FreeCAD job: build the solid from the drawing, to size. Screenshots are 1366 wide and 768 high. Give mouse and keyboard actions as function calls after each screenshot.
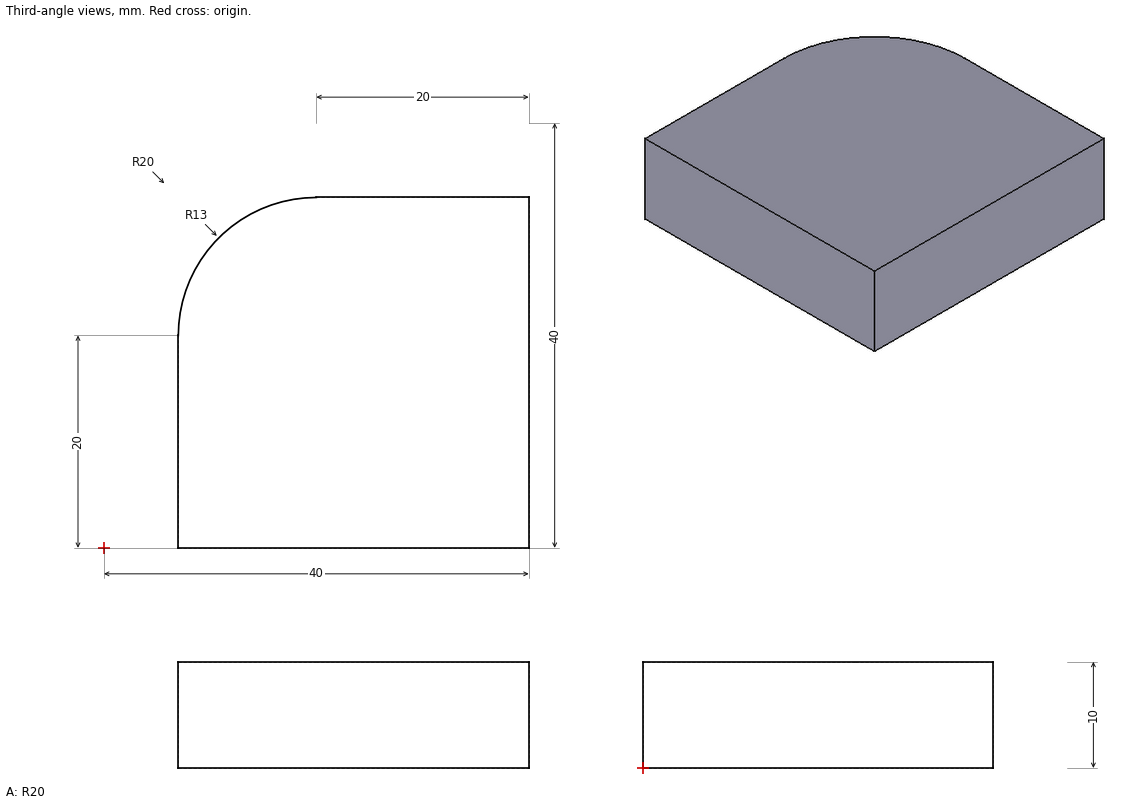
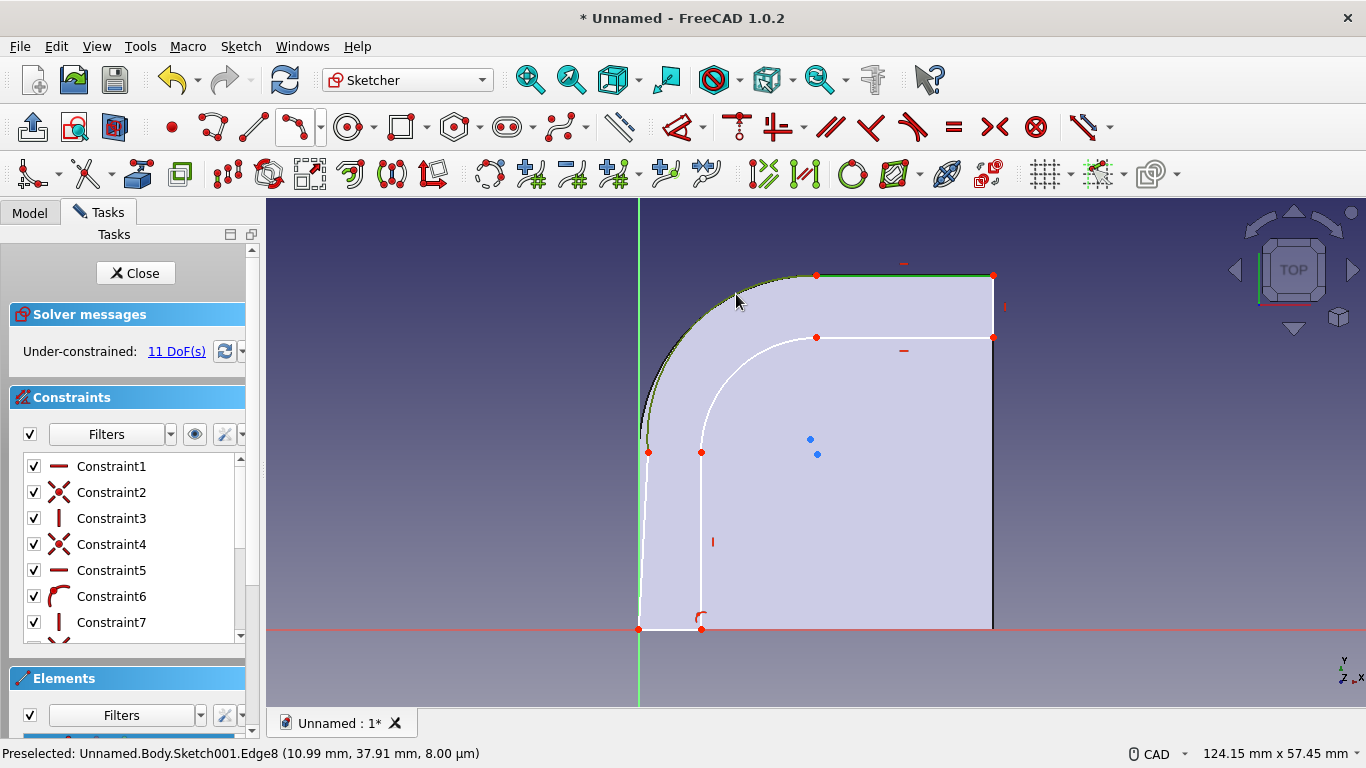
key(t)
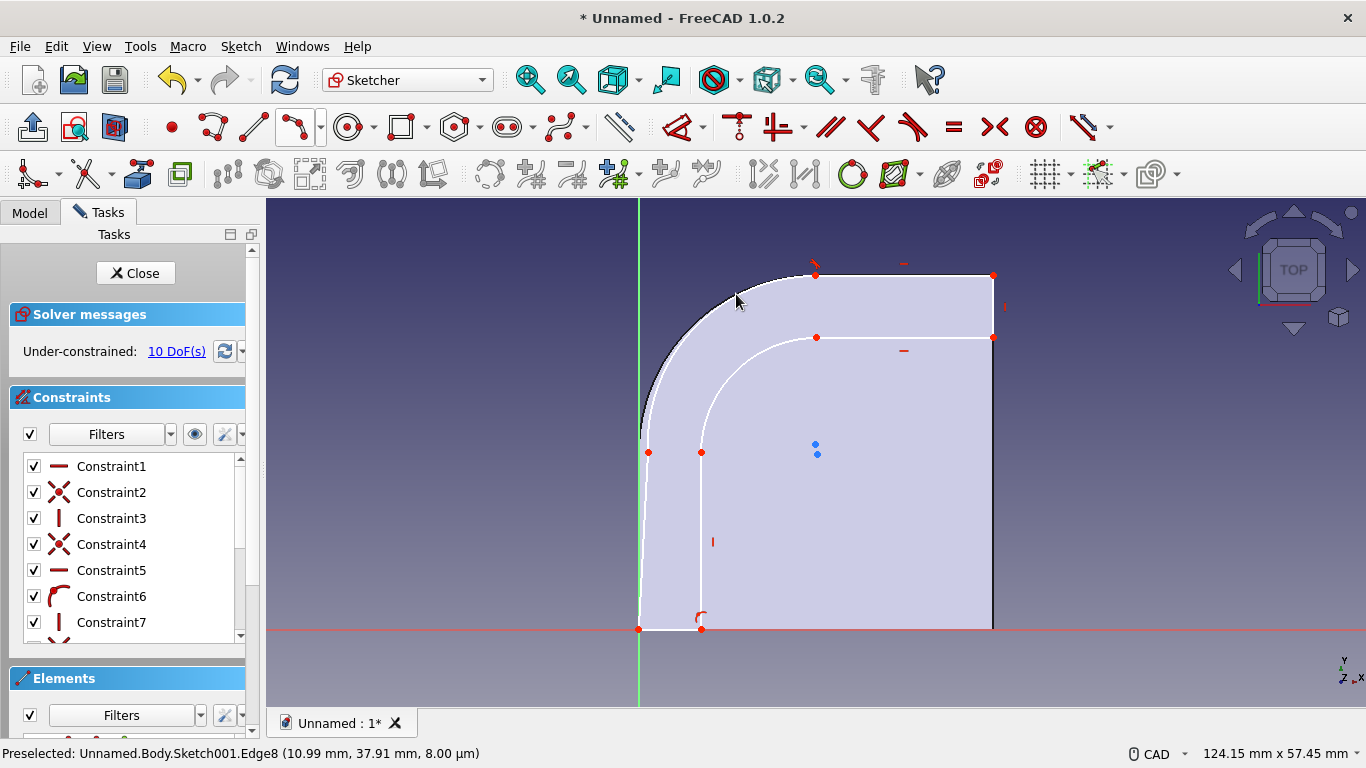
click(940, 338)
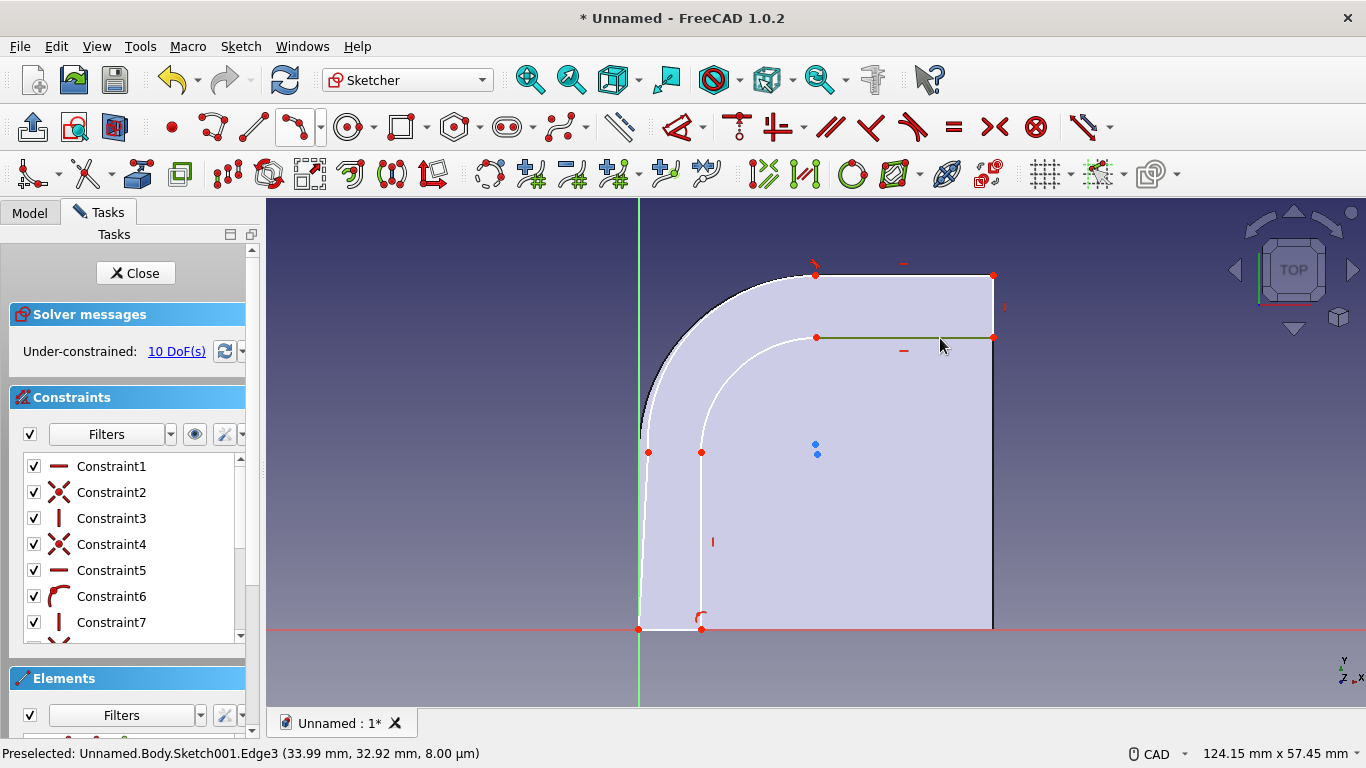
click(764, 351)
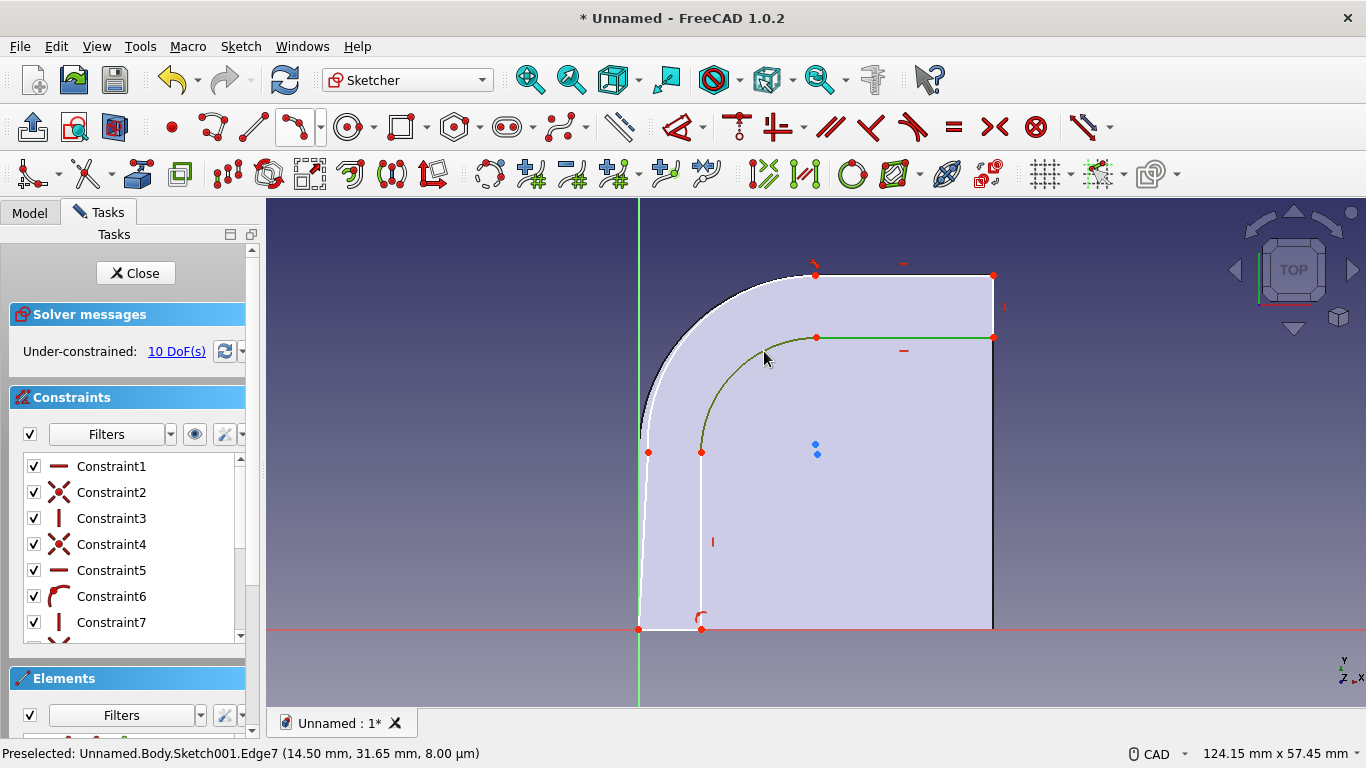
click(913, 128)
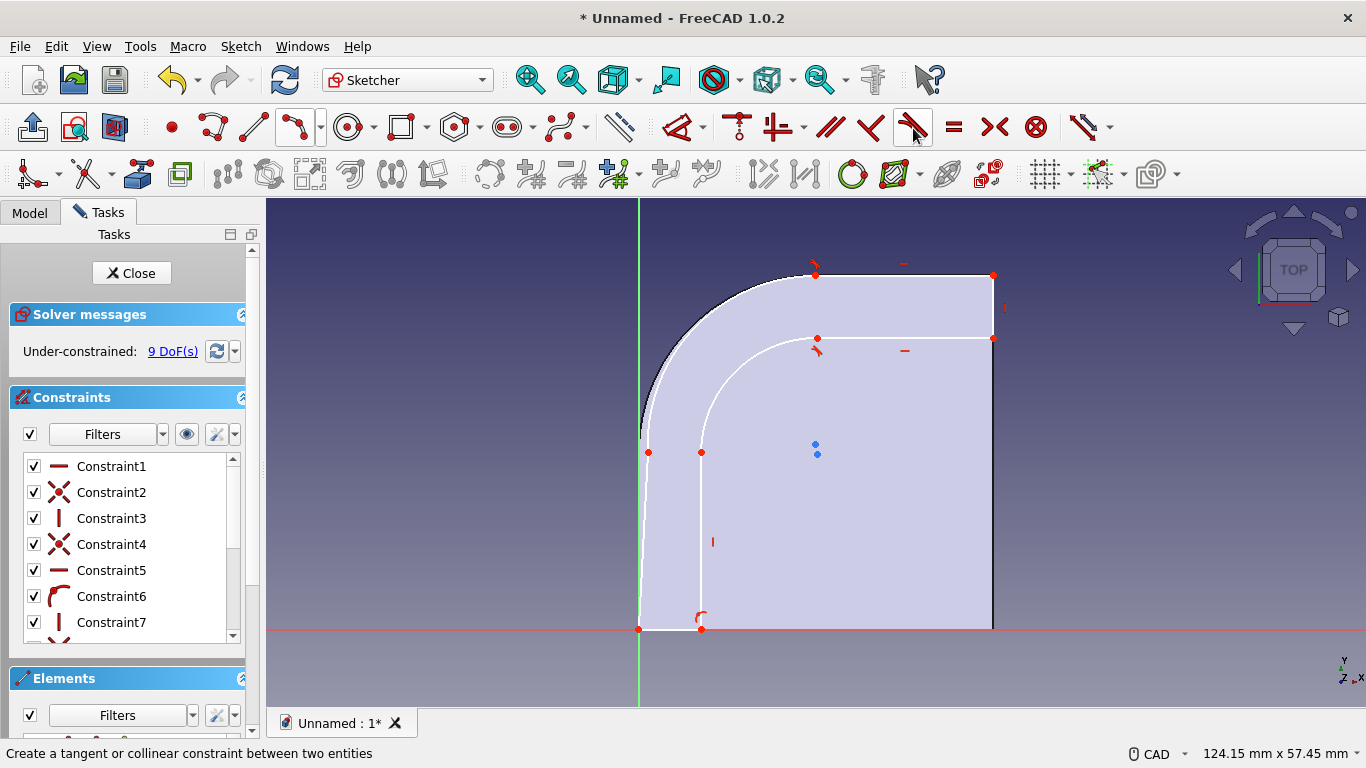
click(701, 506)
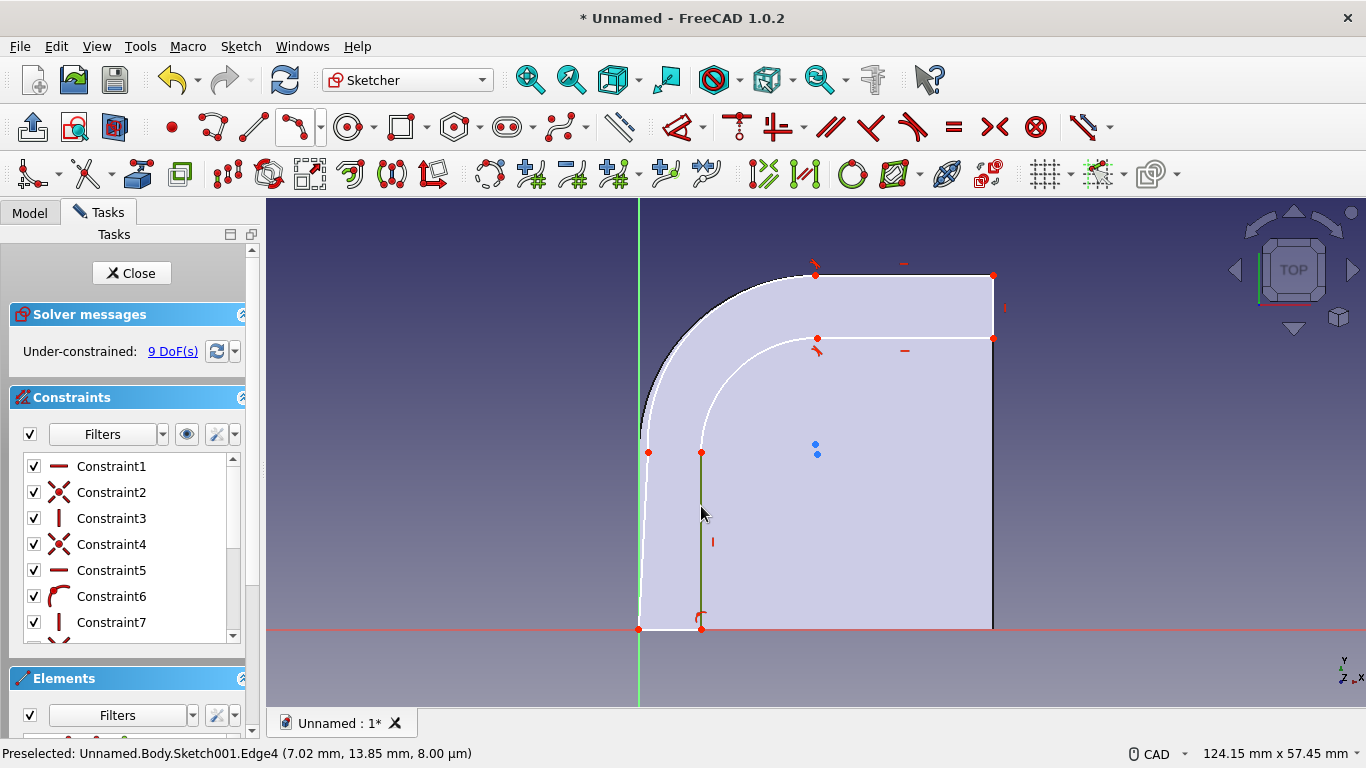
click(765, 351)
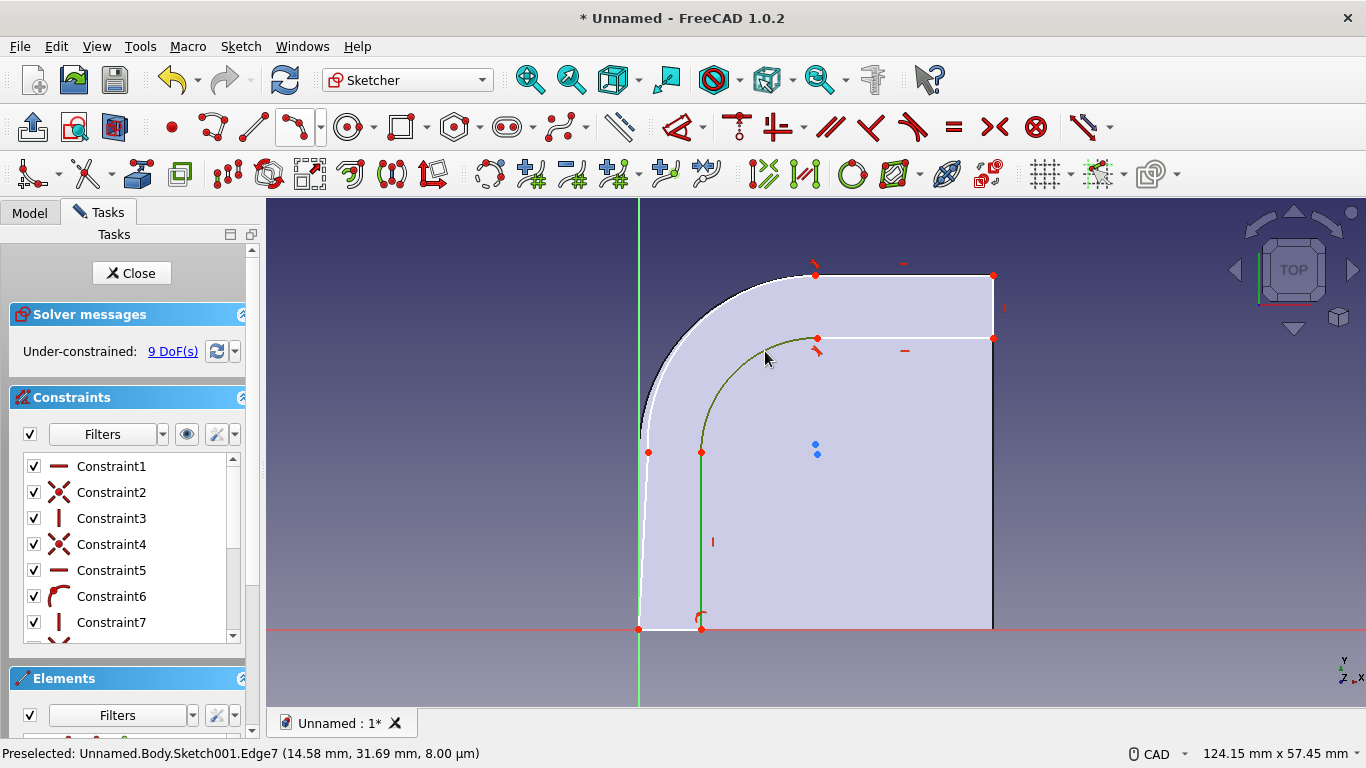
click(913, 128)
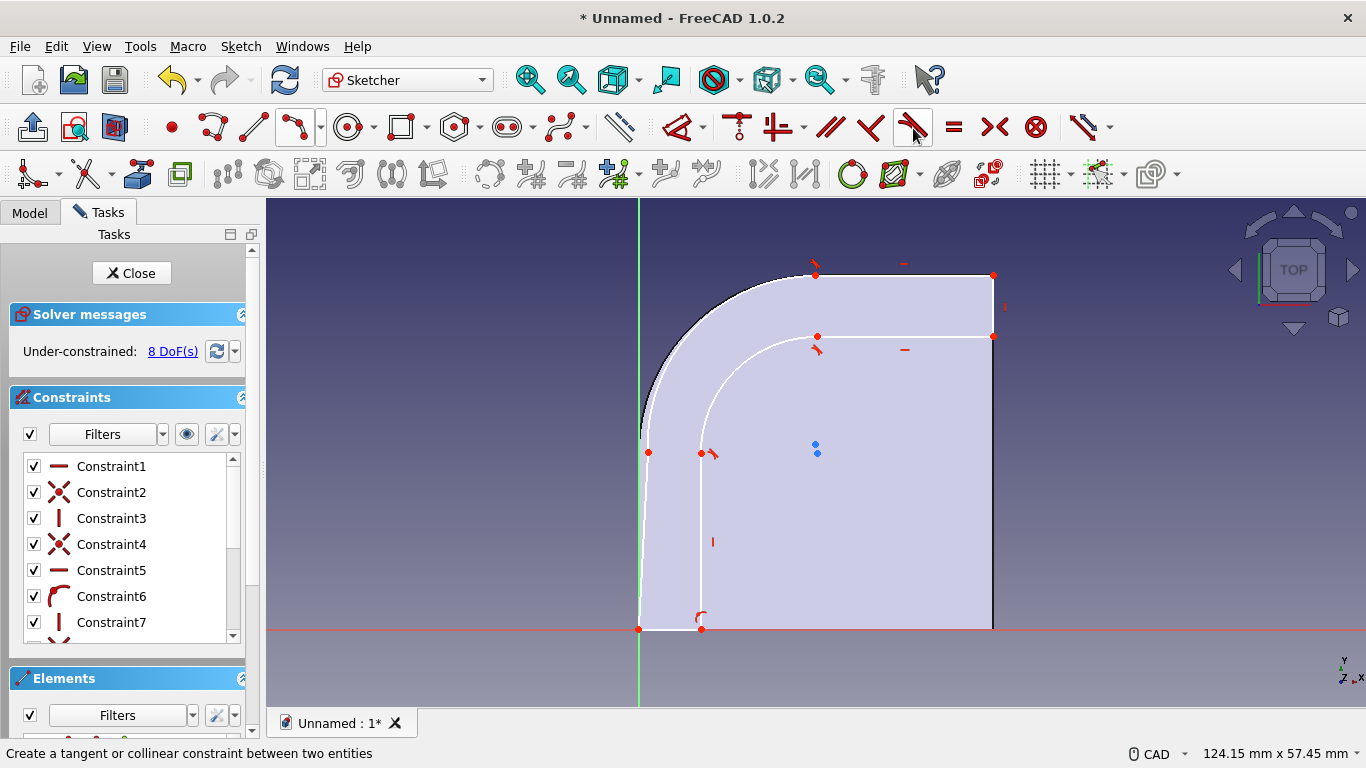
click(642, 577)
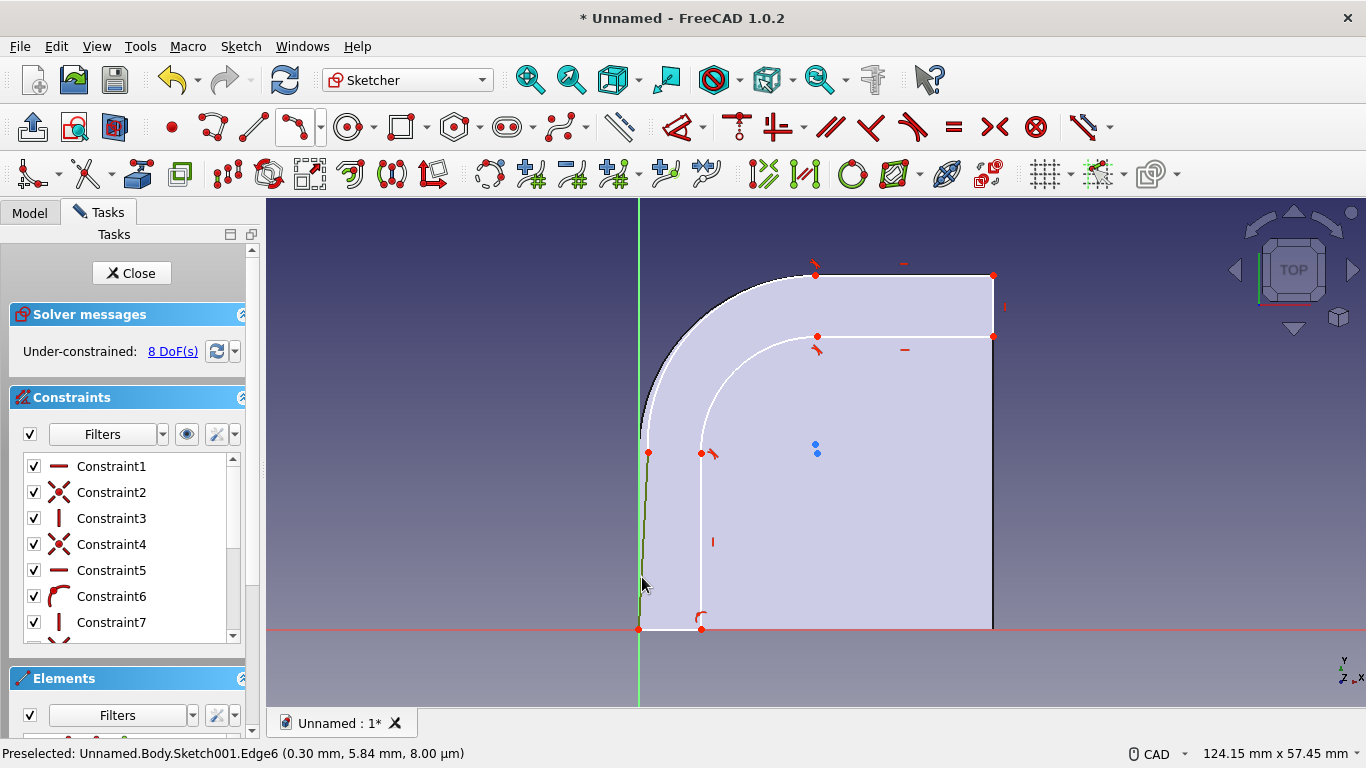
click(737, 296)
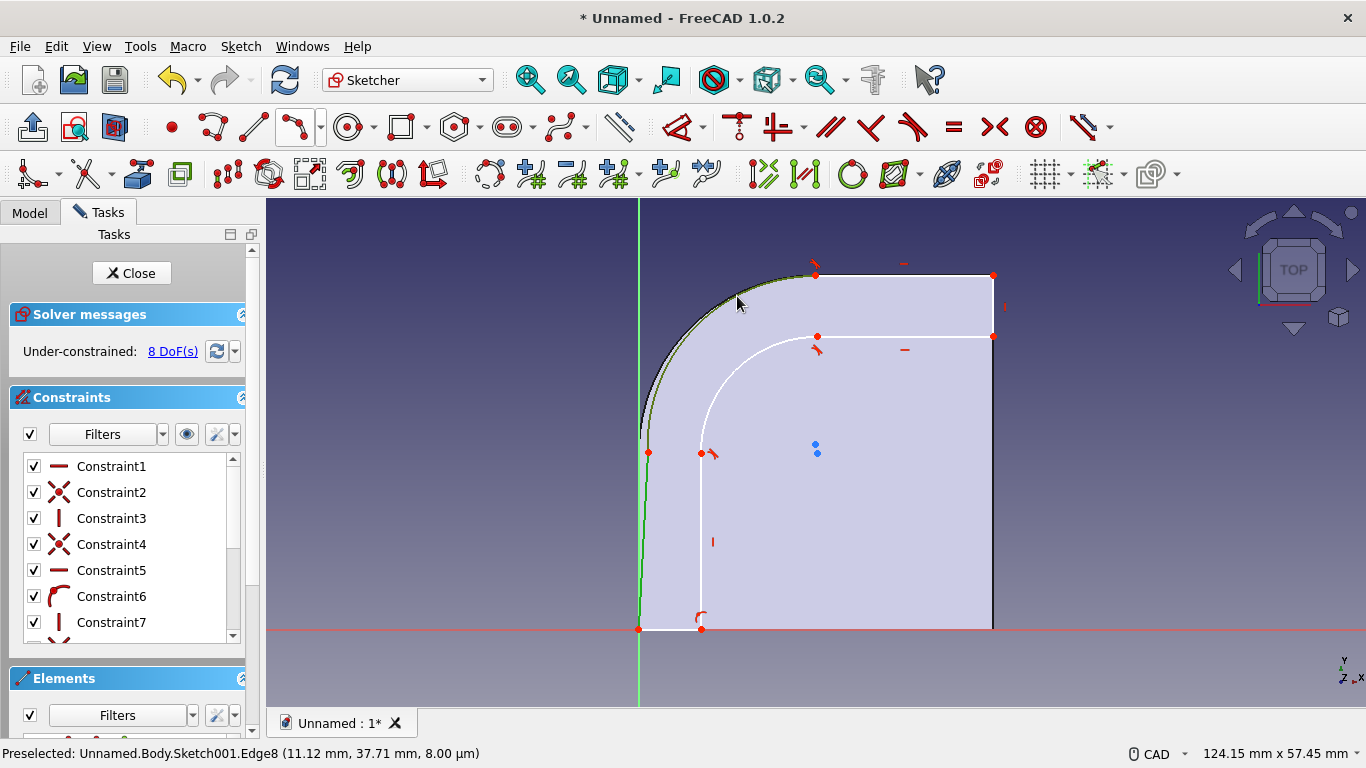
click(913, 128)